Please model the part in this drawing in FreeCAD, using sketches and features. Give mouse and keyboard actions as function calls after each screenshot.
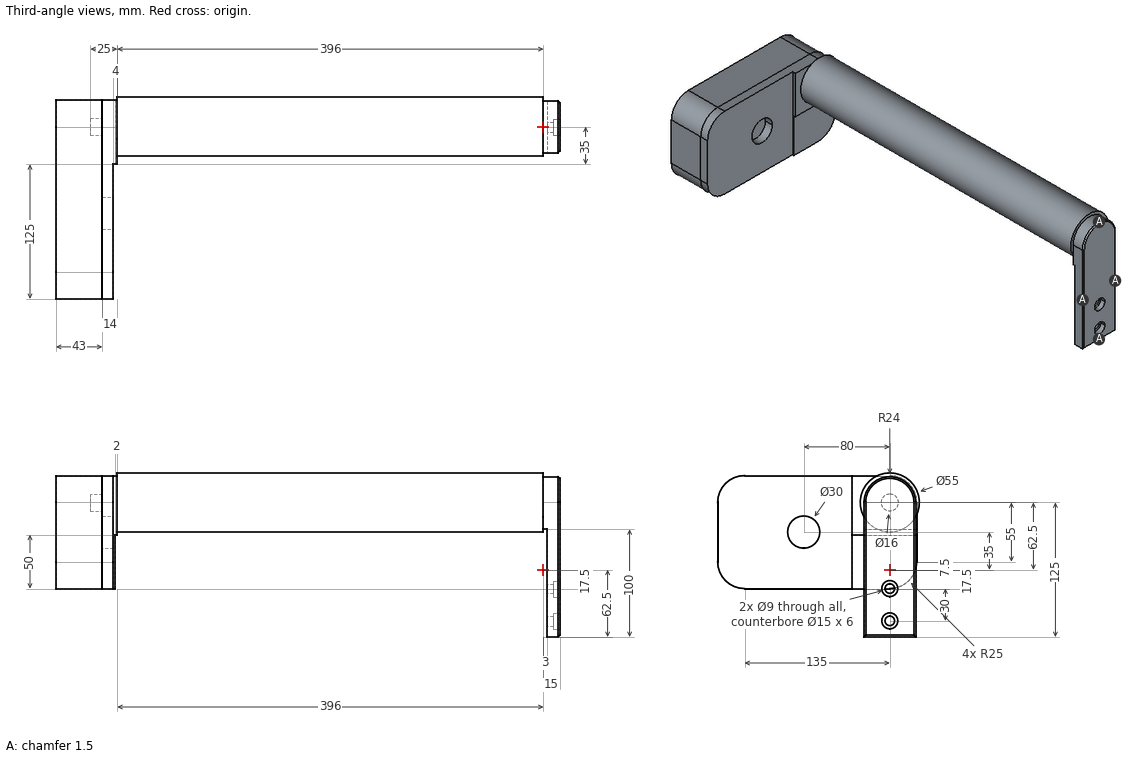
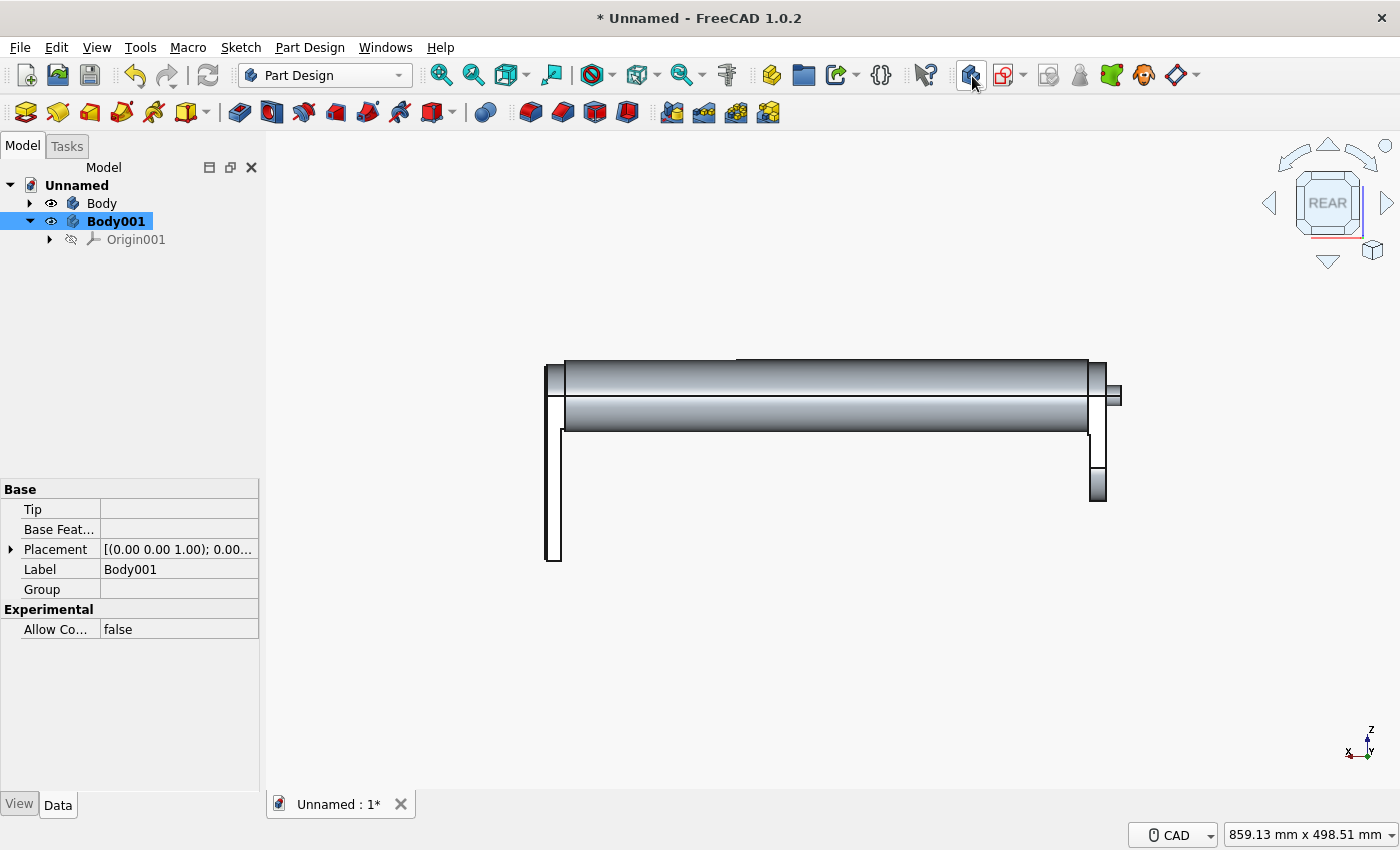
click(50, 239)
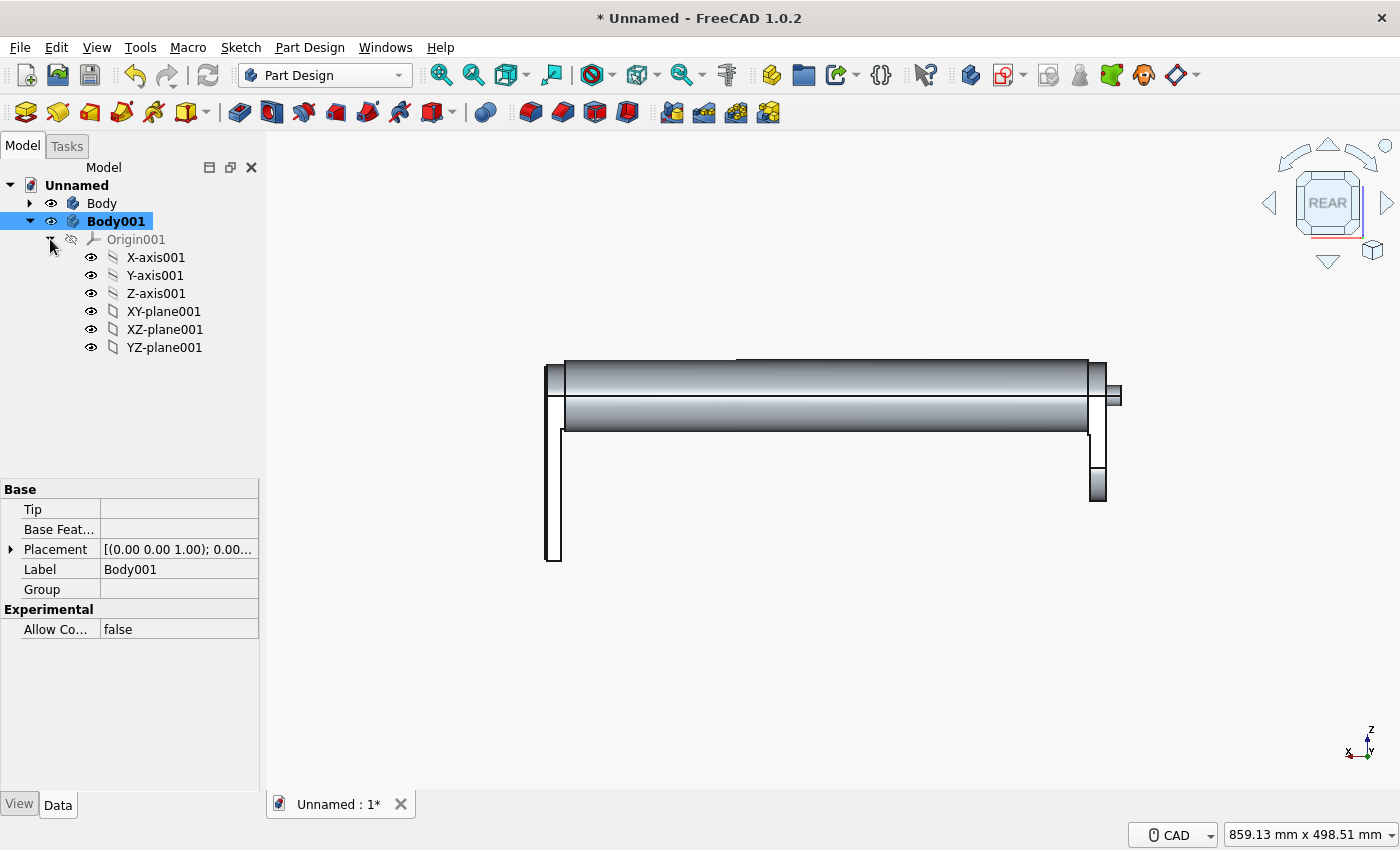
click(136, 347)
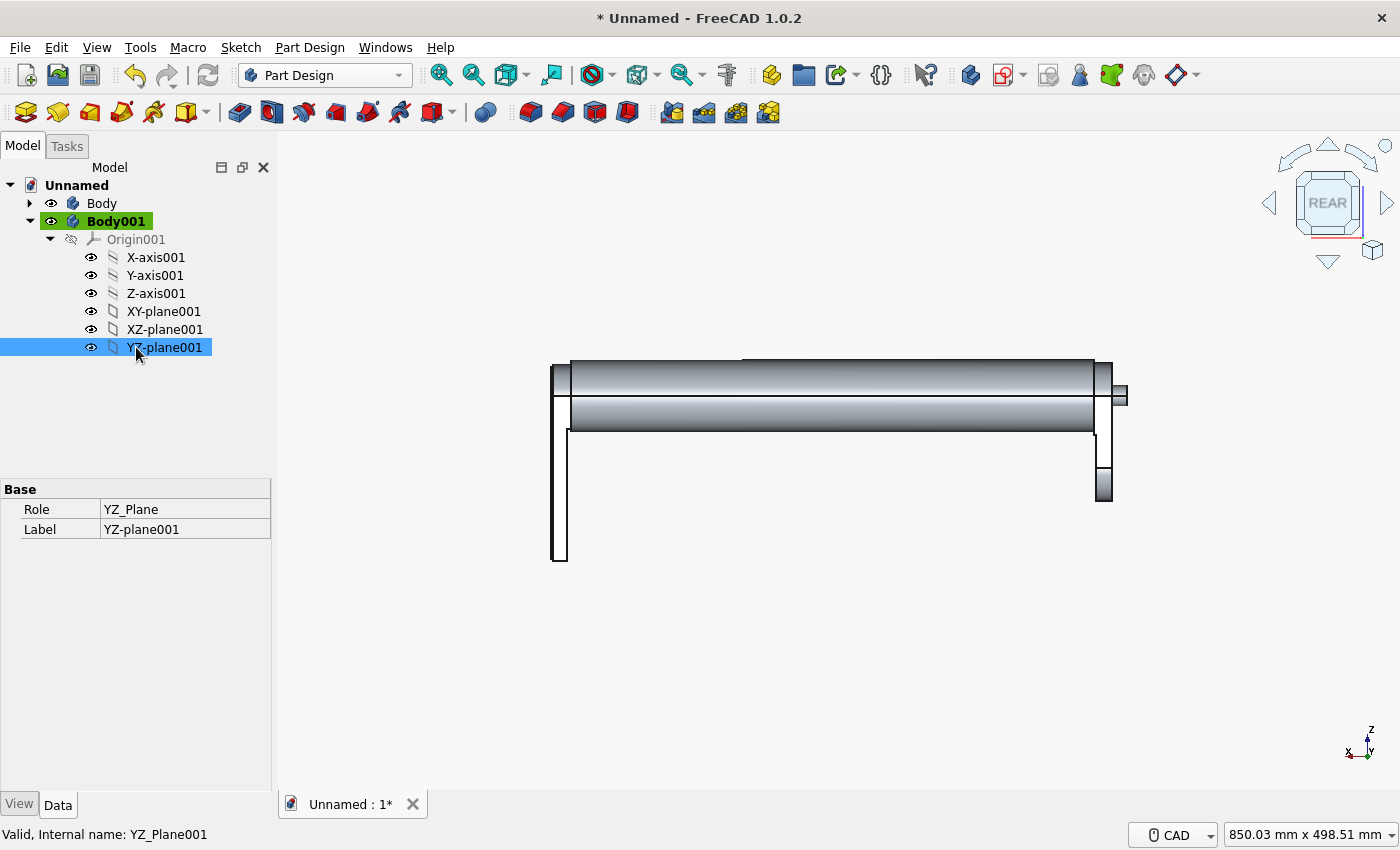
click(1176, 76)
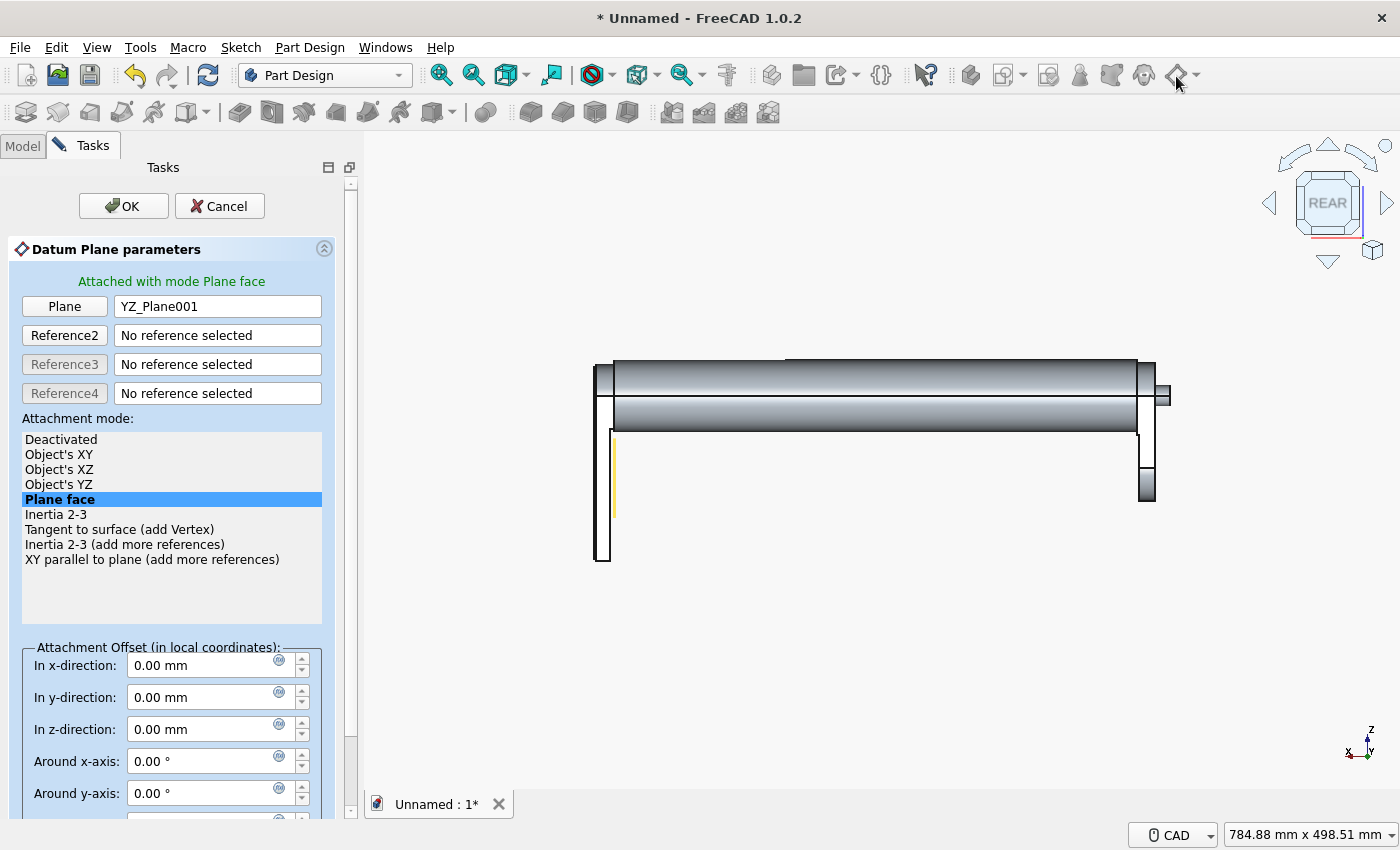
triple_click(210, 729)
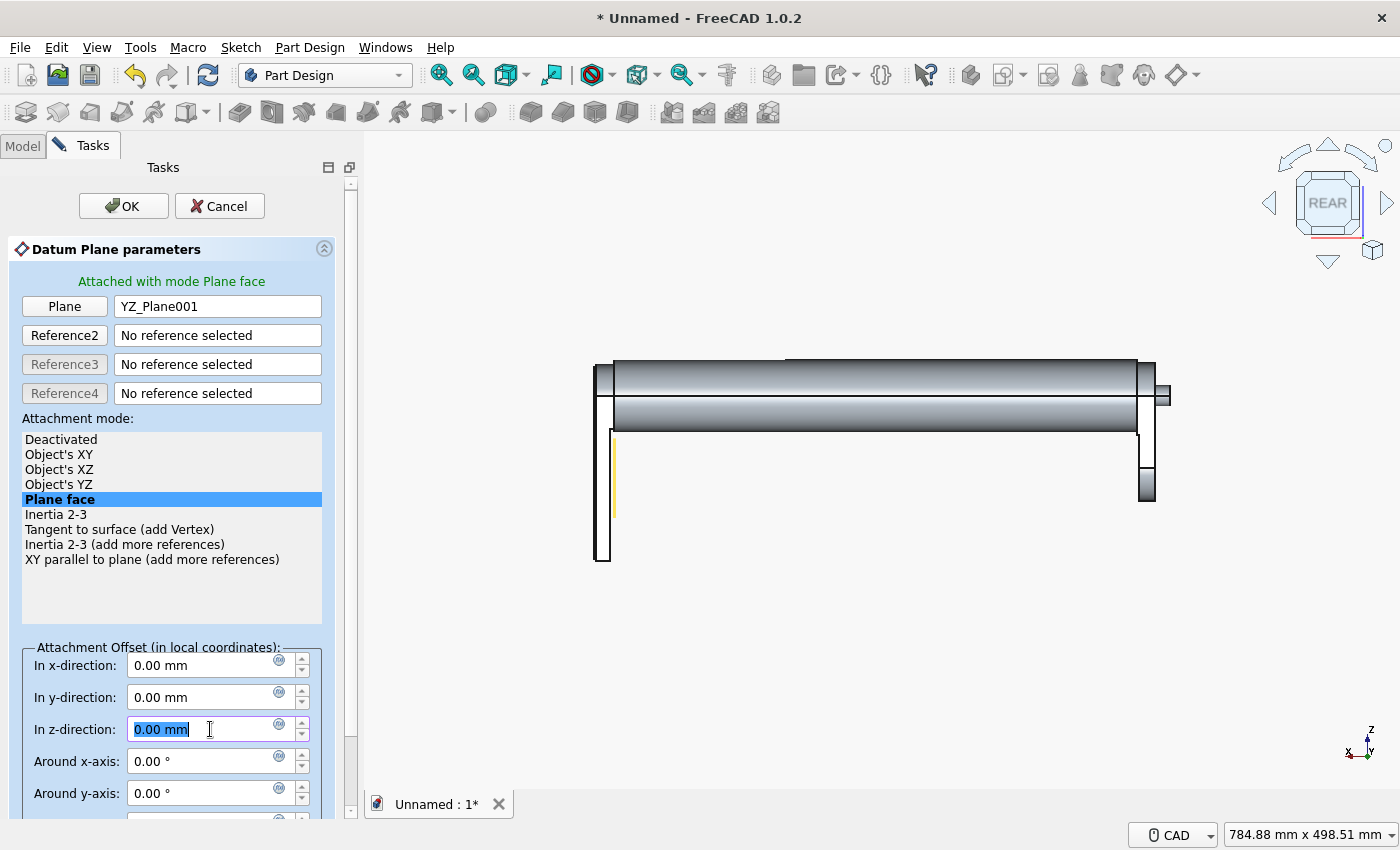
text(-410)
key(Tab)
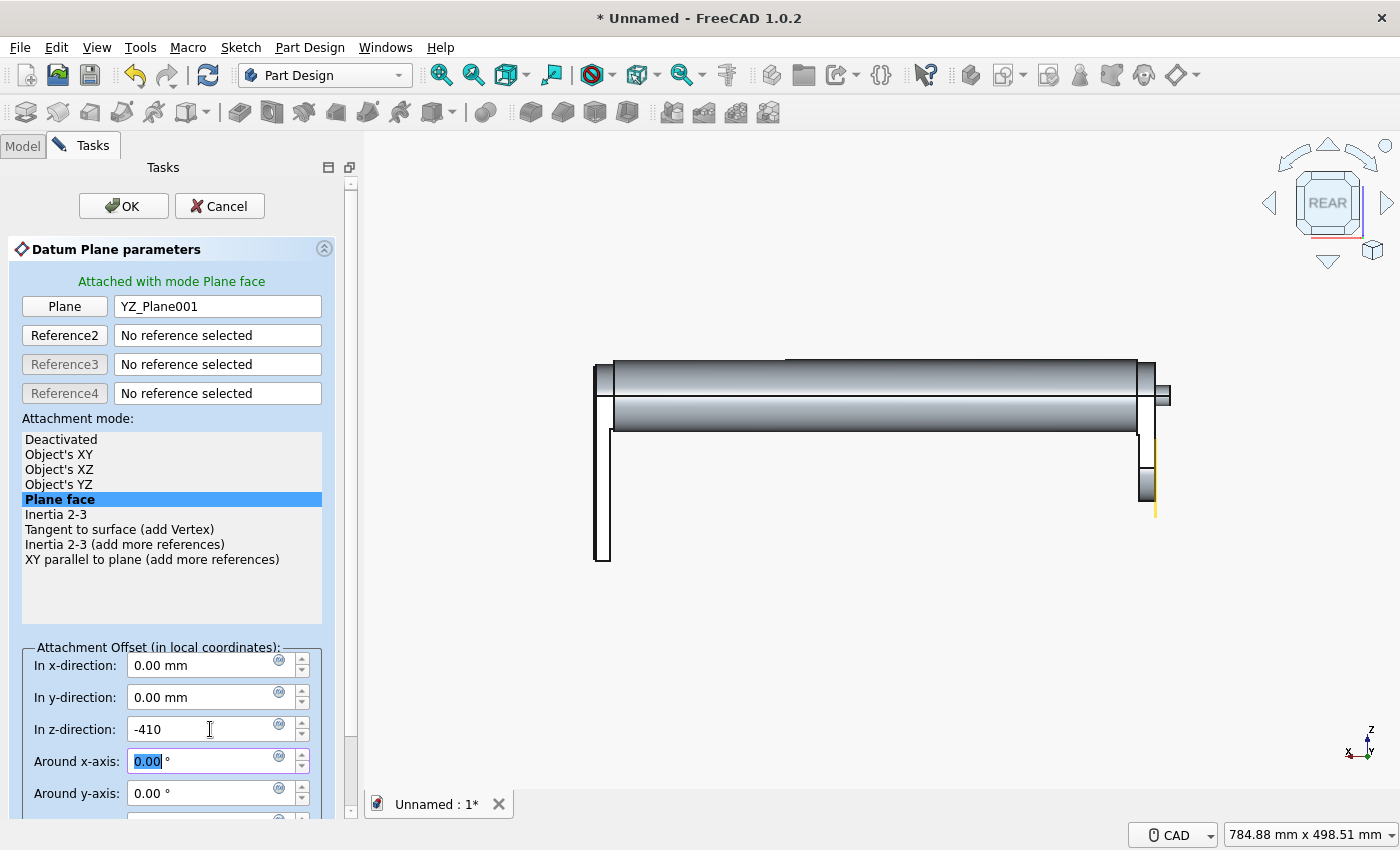
click(124, 206)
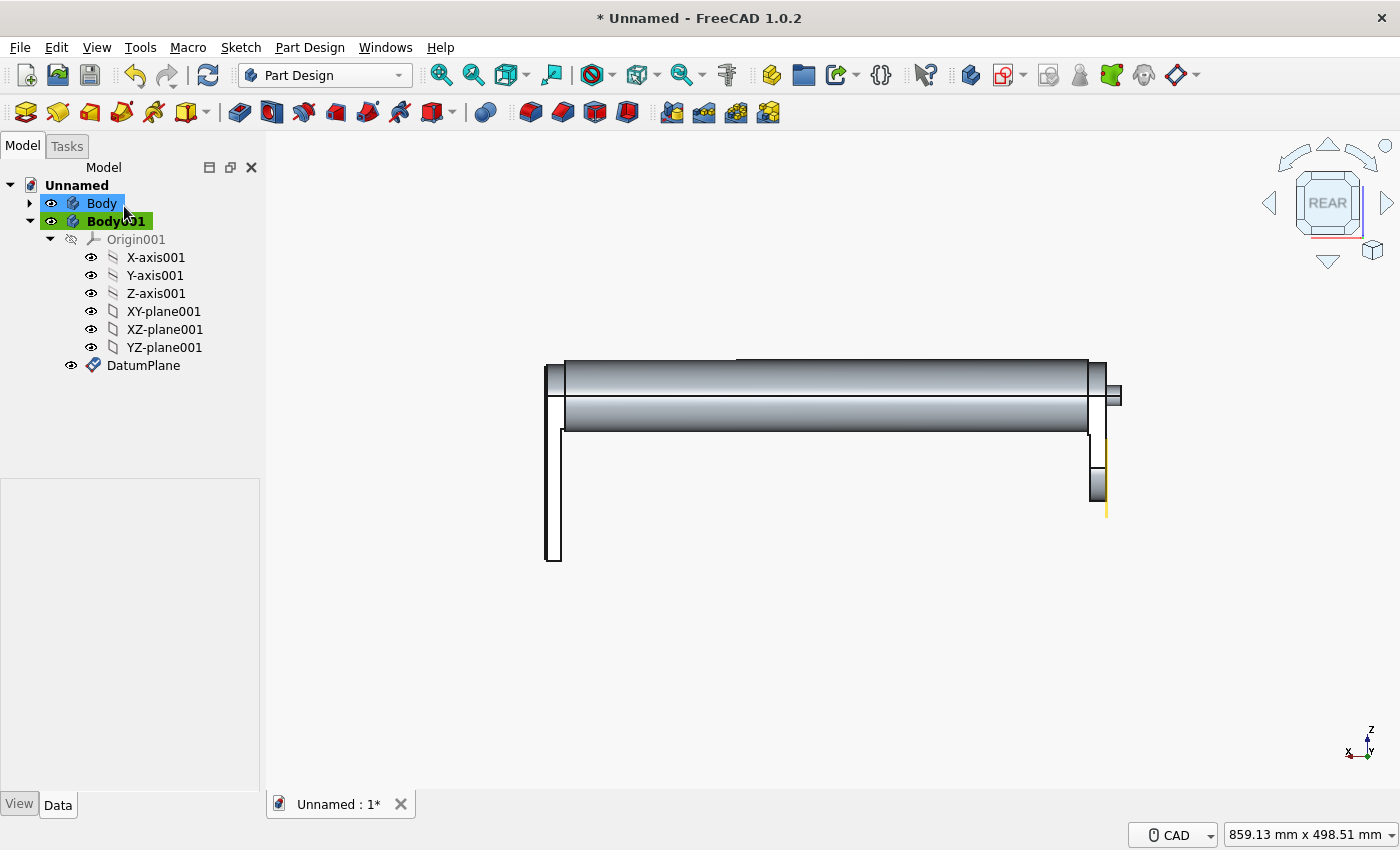
click(116, 365)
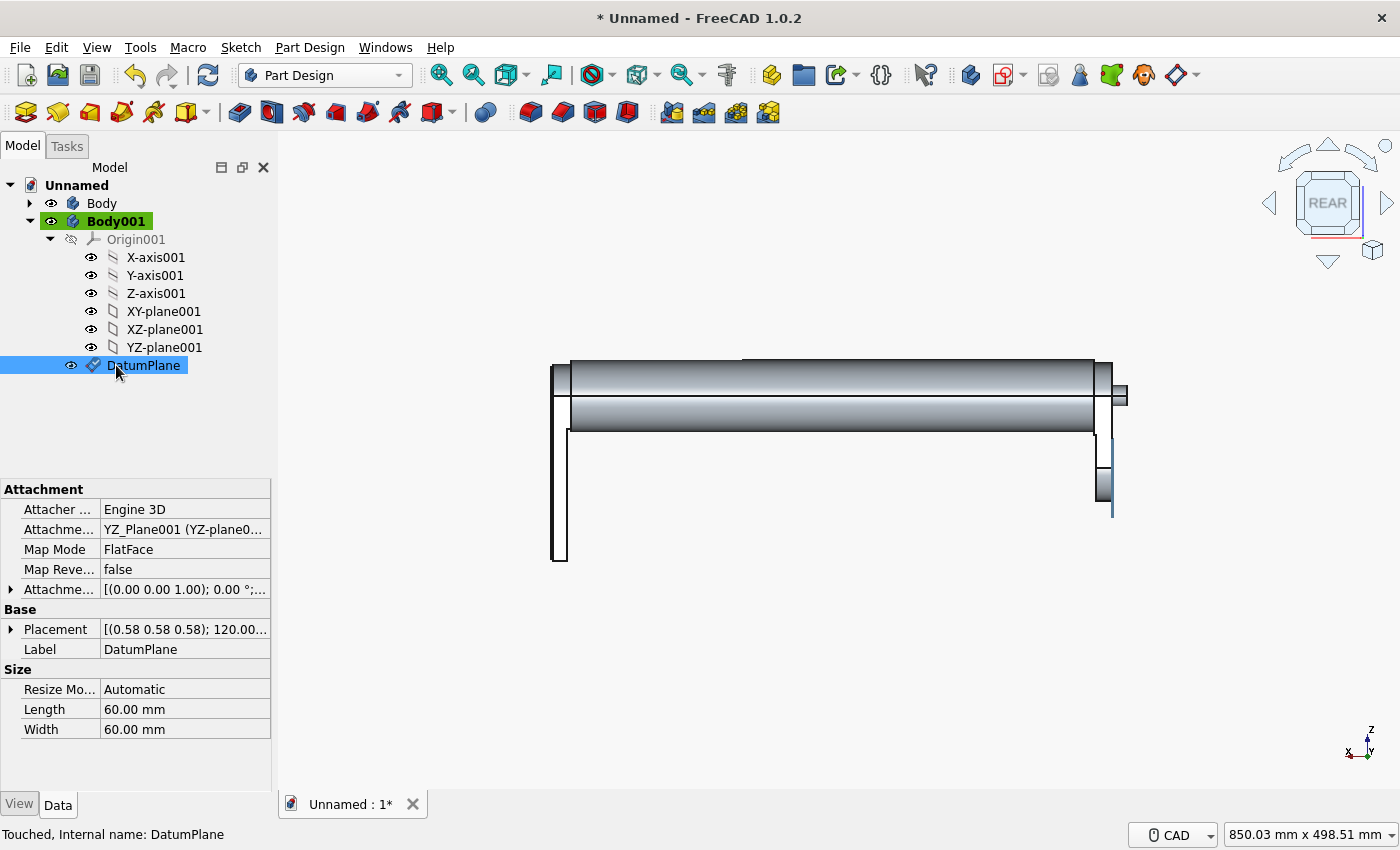
click(1004, 76)